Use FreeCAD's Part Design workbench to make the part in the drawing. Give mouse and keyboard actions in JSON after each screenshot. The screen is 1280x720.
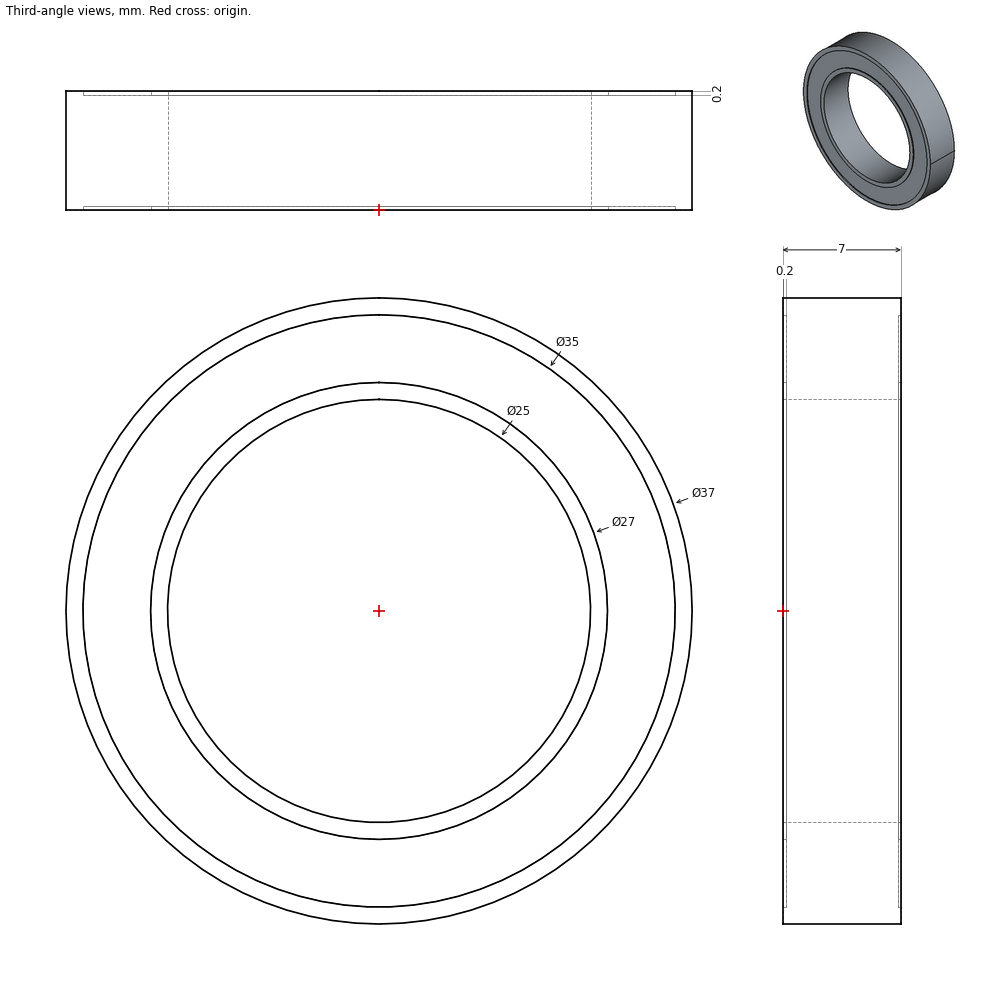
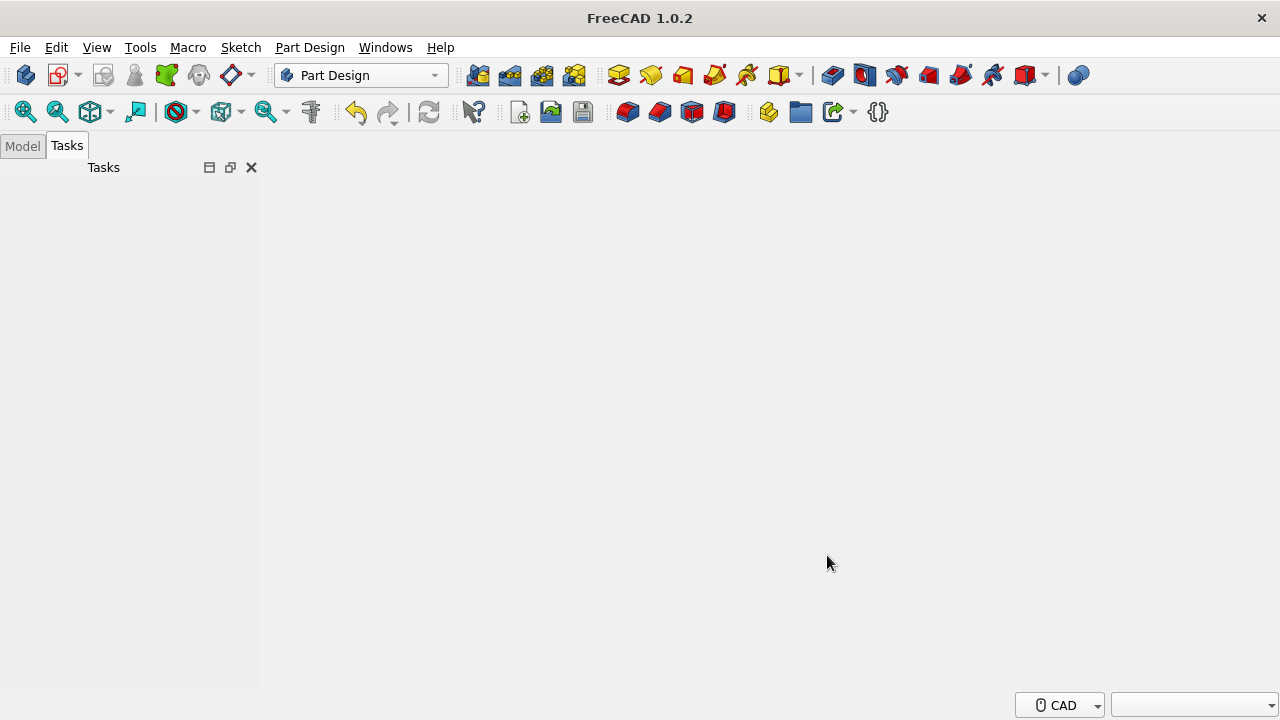
{"action": "key", "text": "ctrl+n"}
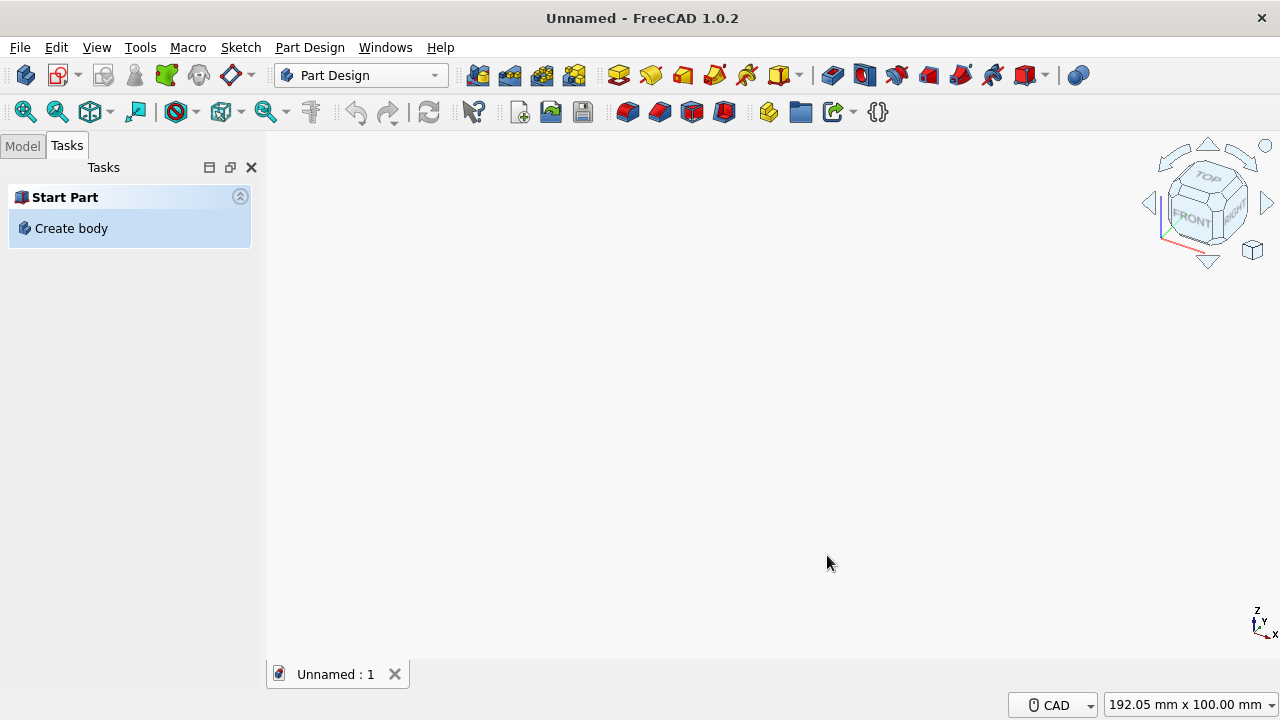
{"action": "left_click", "coordinate": [58, 76]}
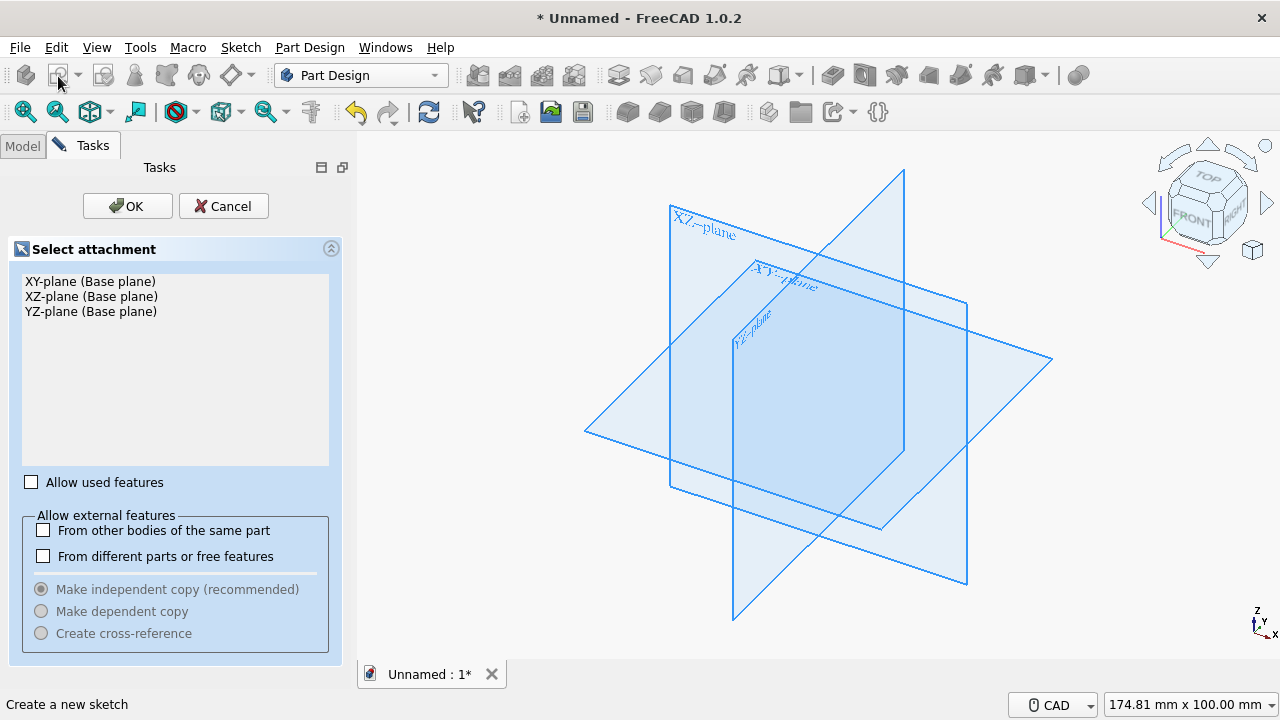
{"action": "left_click", "coordinate": [82, 296]}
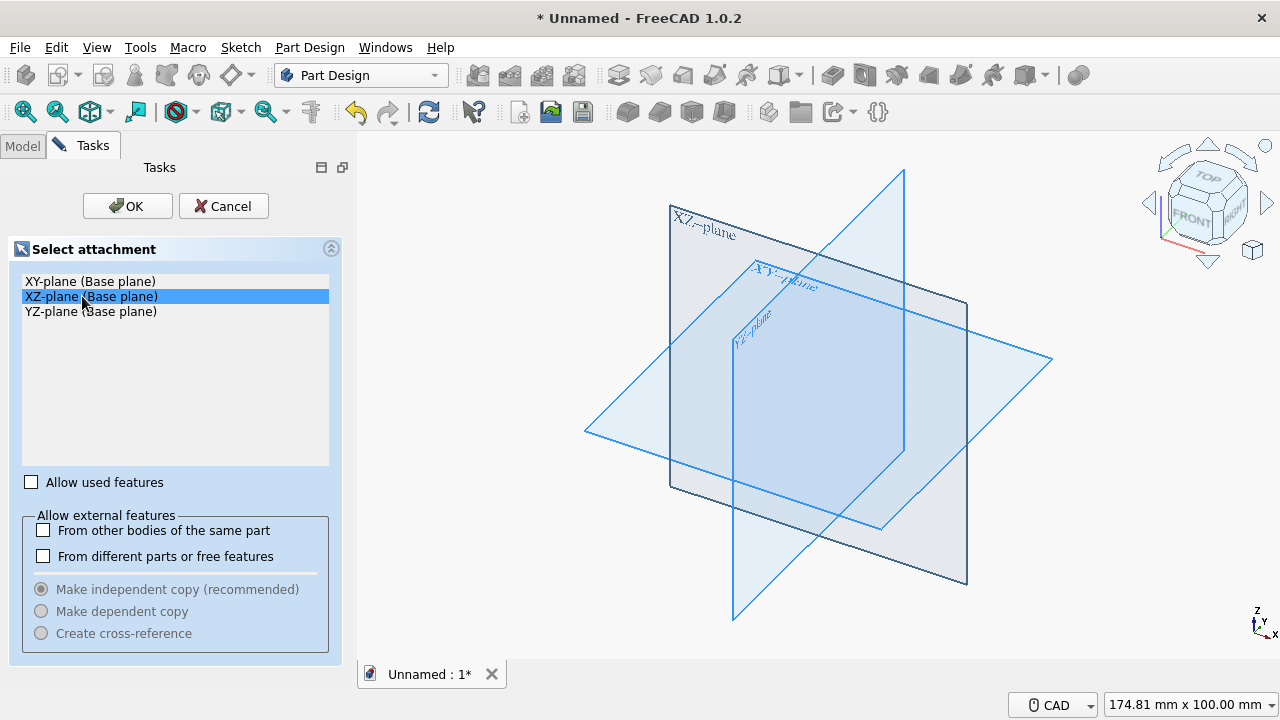
{"action": "left_click", "coordinate": [128, 206]}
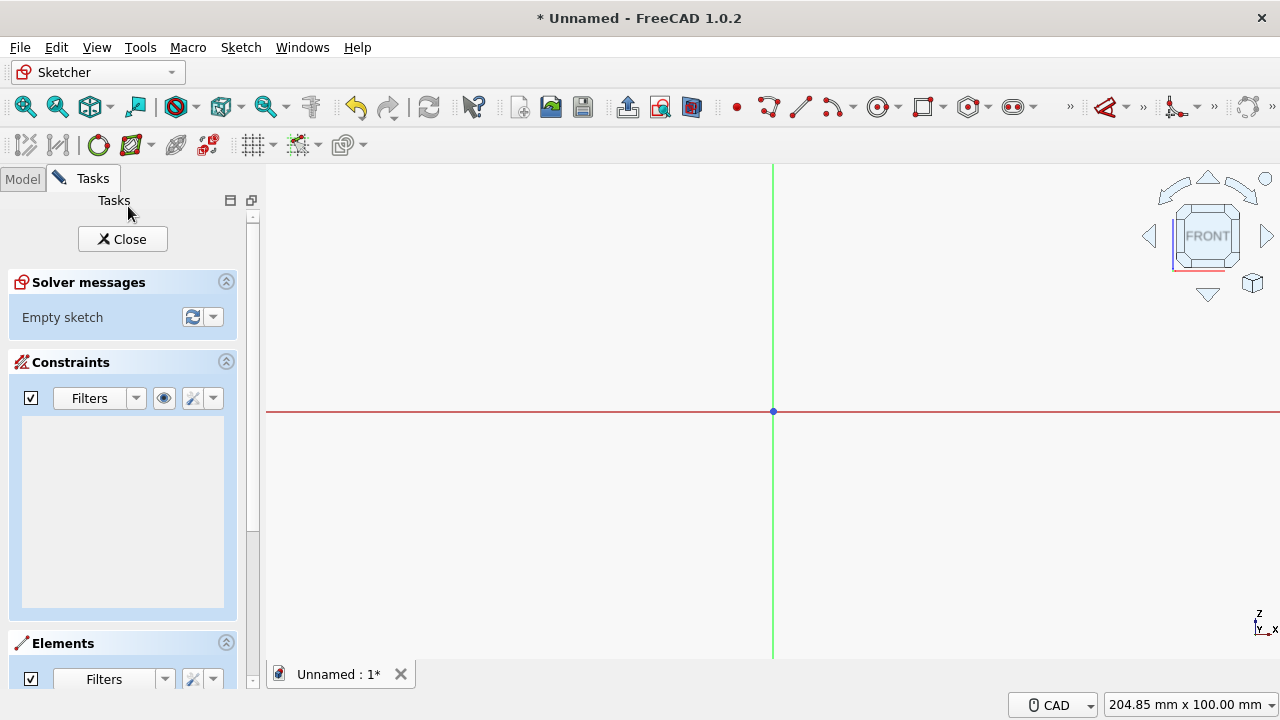
{"action": "scroll", "coordinate": [856, 412], "scroll_direction": "up", "scroll_amount": 3}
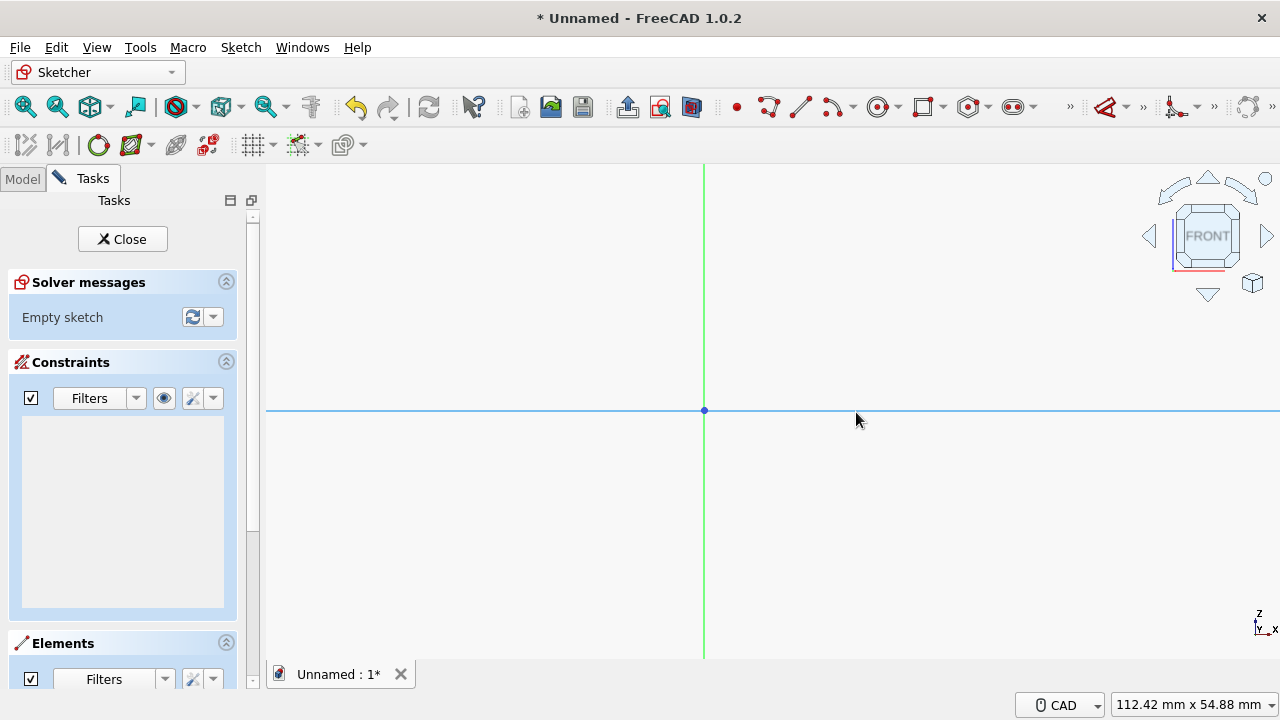
{"action": "key", "text": "g c"}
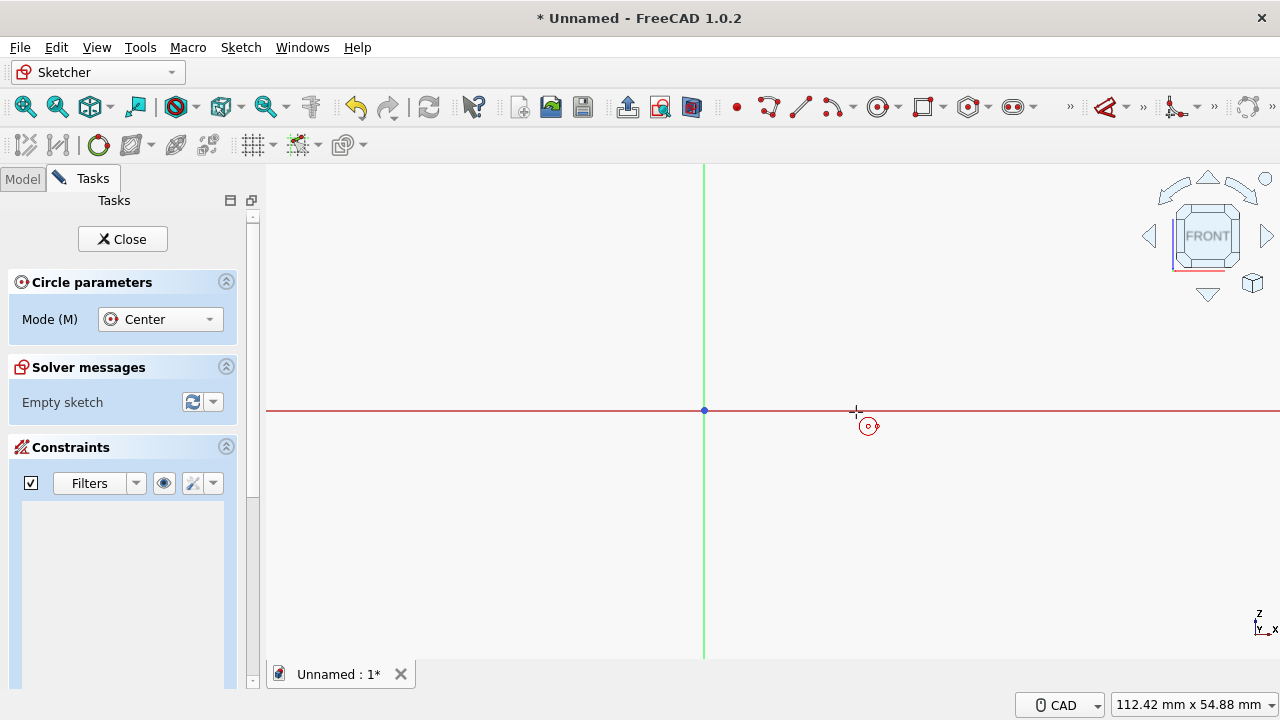
{"action": "left_click", "coordinate": [704, 411]}
{"action": "mouse_move", "coordinate": [822, 293]}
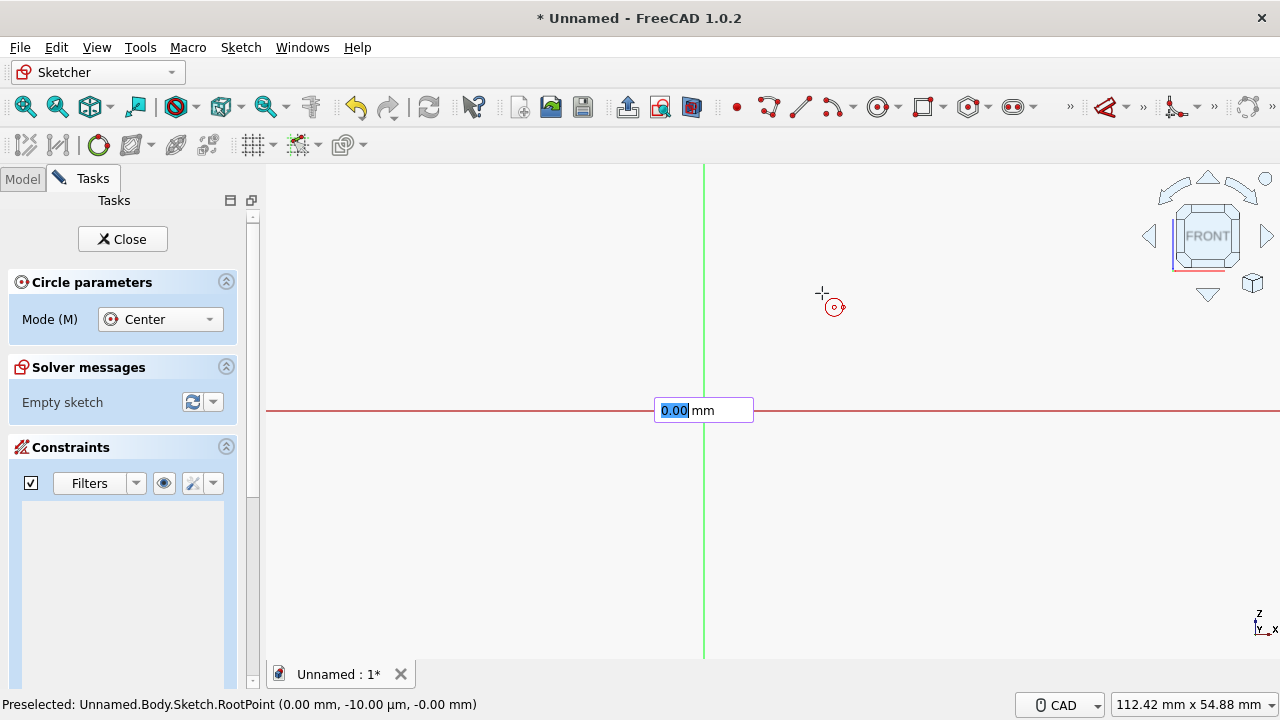
{"action": "type", "text": "37"}
{"action": "key", "text": "Return"}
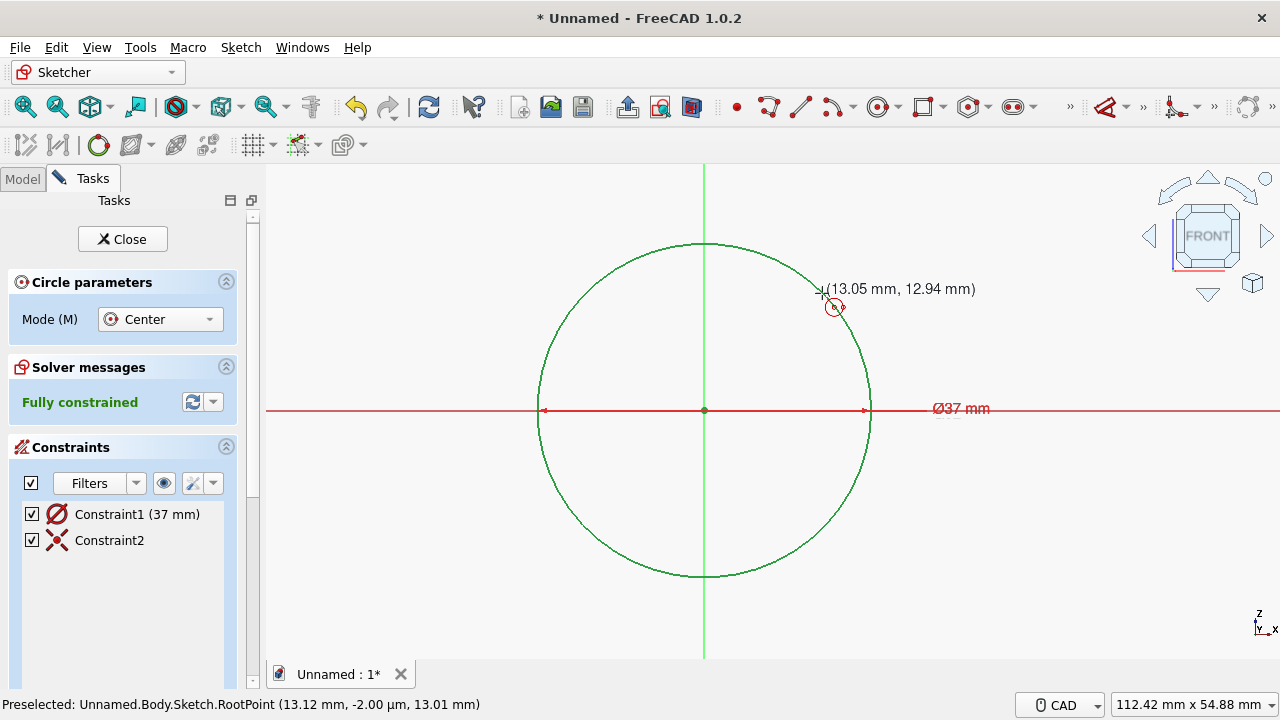
{"action": "left_click", "coordinate": [704, 411]}
{"action": "mouse_move", "coordinate": [784, 331]}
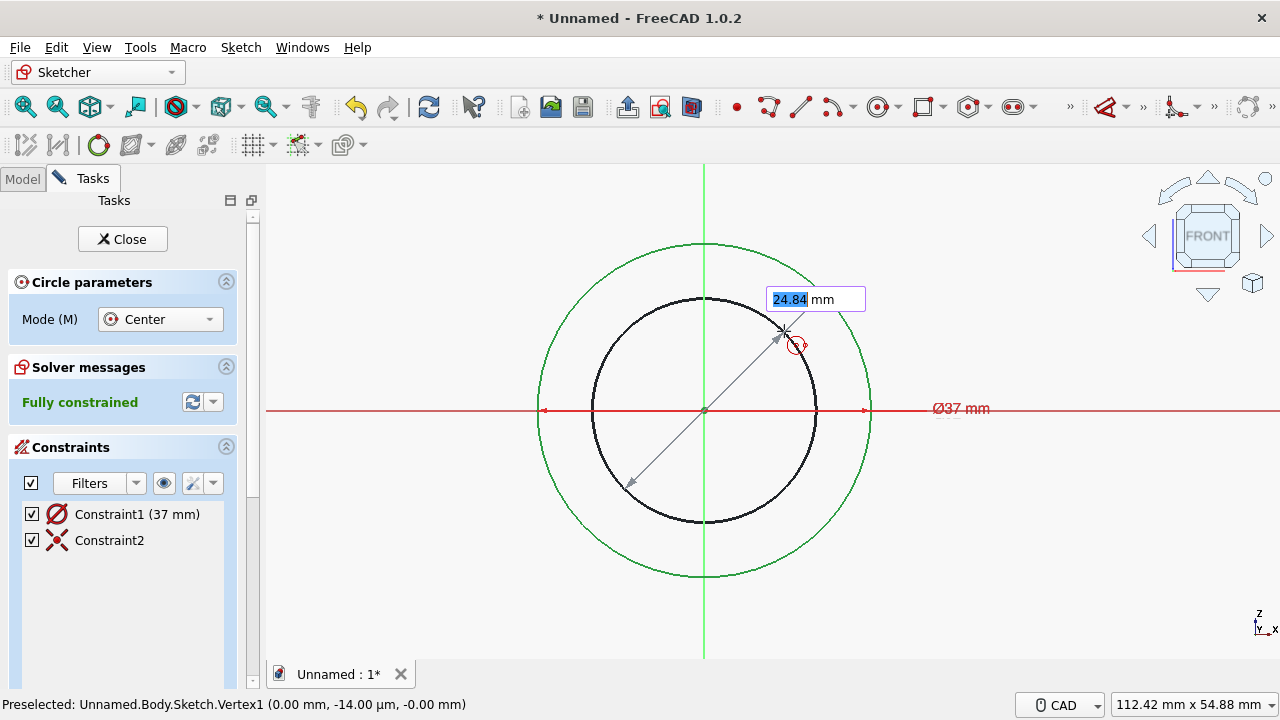
{"action": "type", "text": "25"}
{"action": "key", "text": "Return"}
{"action": "key", "text": "Escape"}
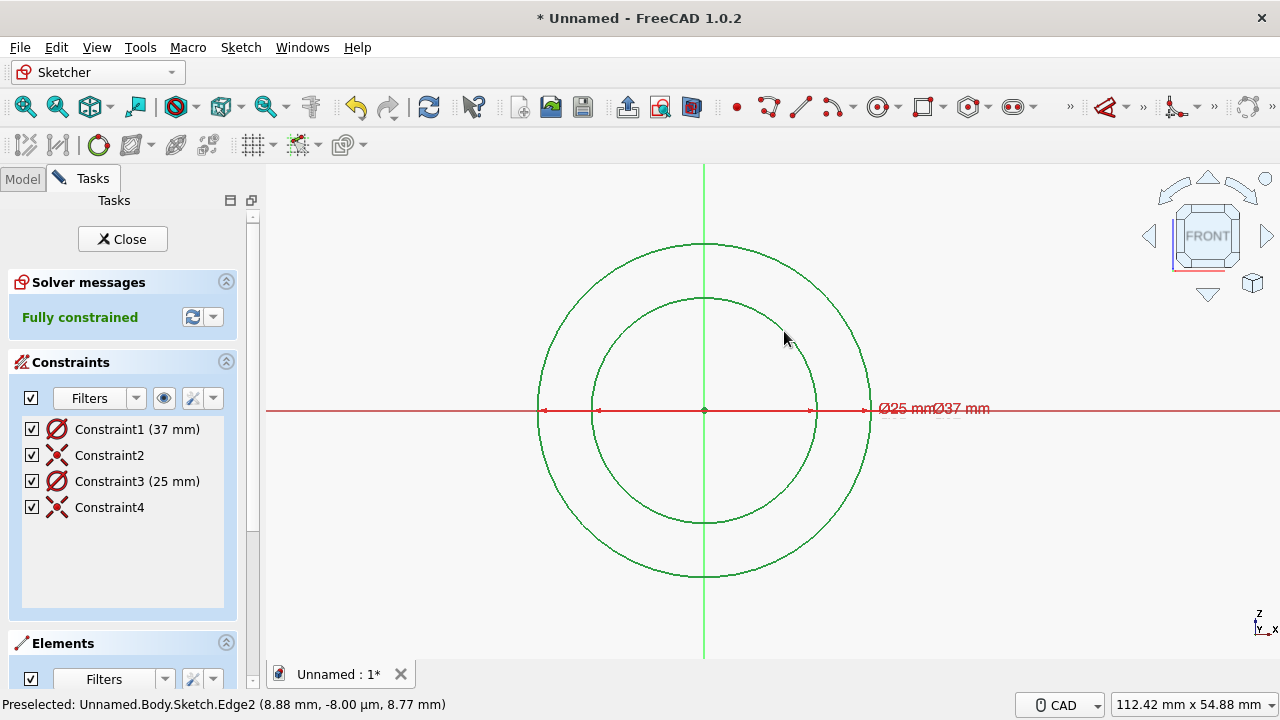
{"action": "left_click", "coordinate": [123, 239]}